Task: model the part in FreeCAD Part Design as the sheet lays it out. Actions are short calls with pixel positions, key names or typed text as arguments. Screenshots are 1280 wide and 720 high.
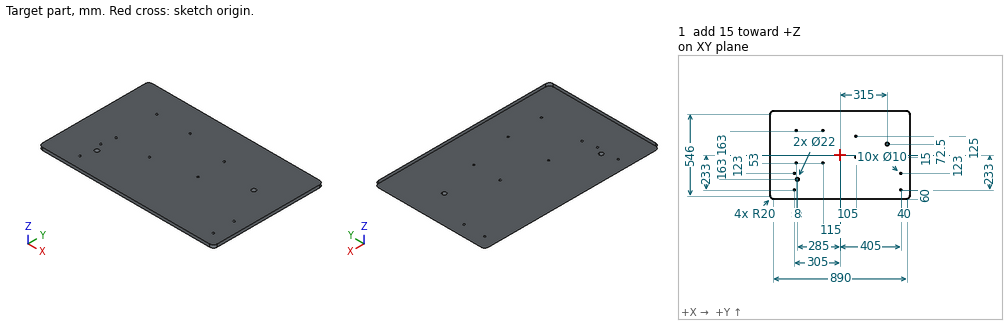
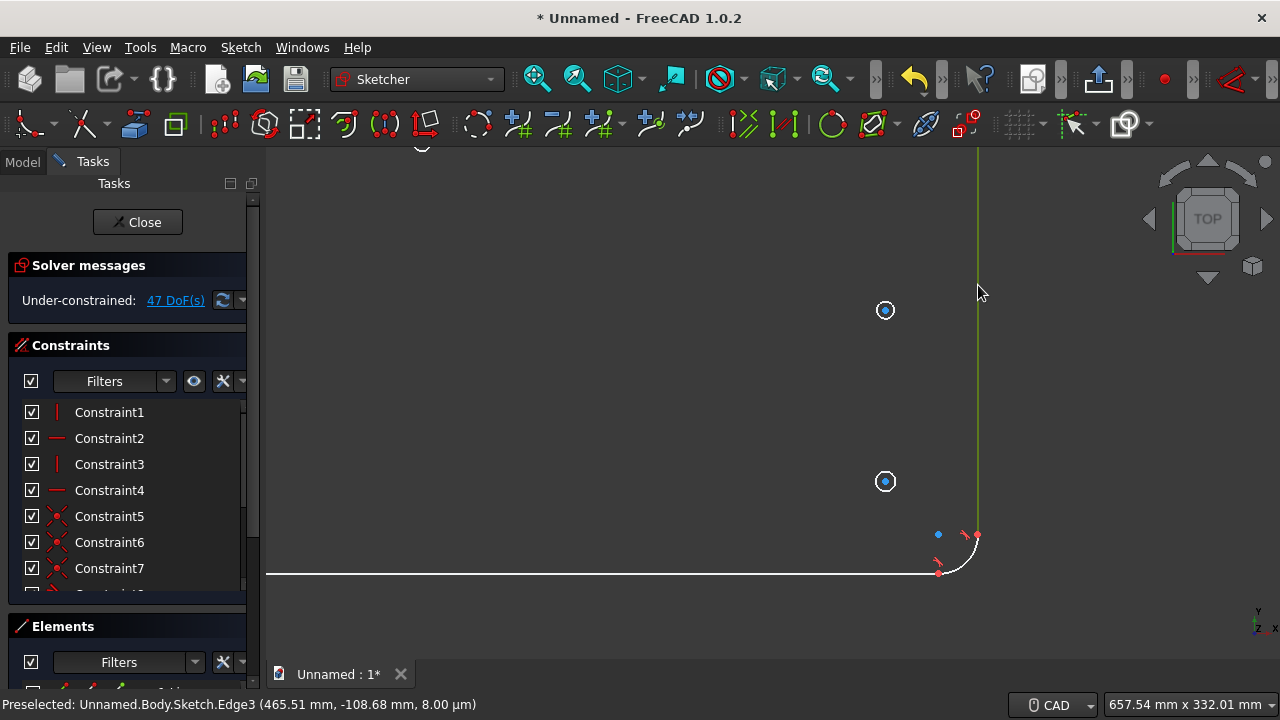
scroll(963, 569, down, 5)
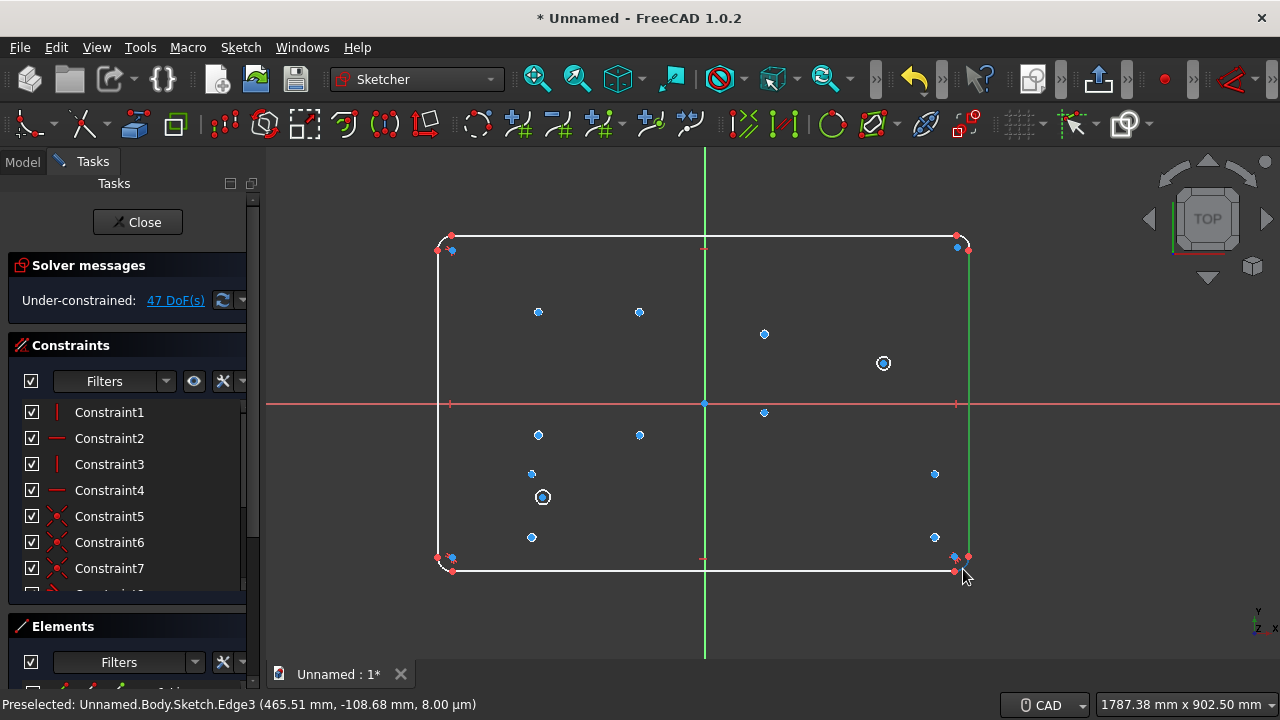
scroll(969, 244, up, 4)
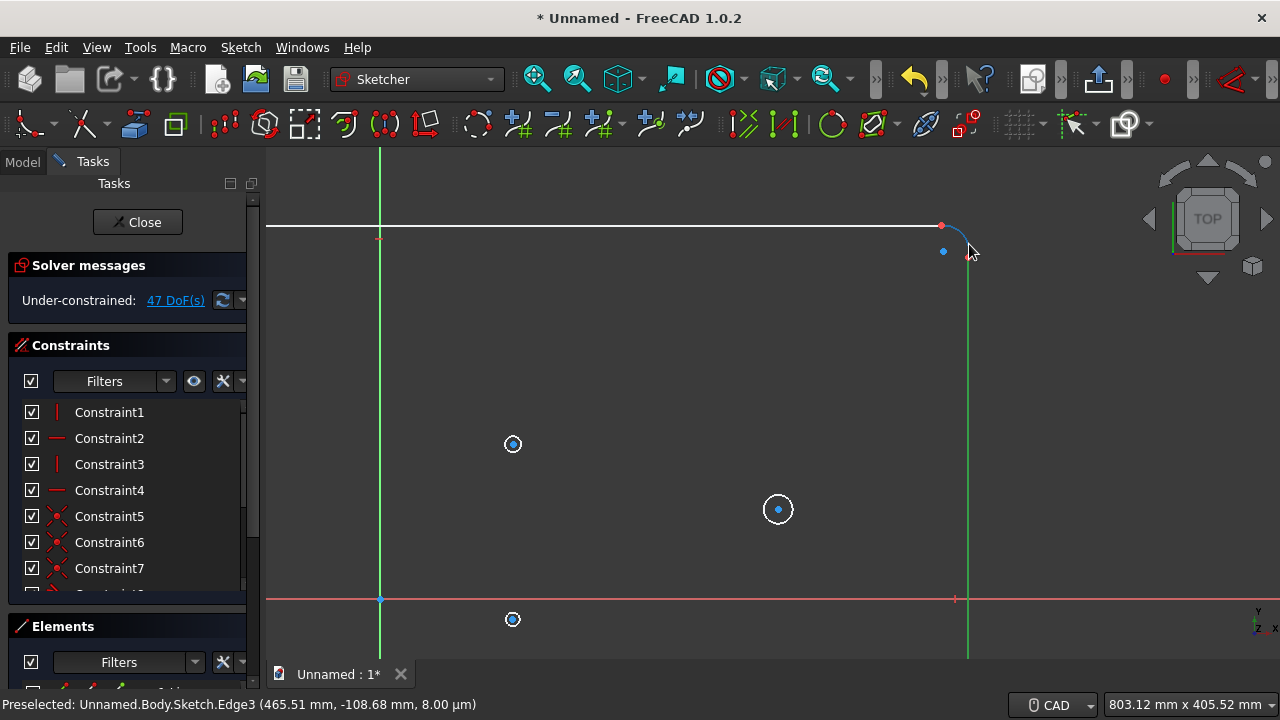
click(968, 243)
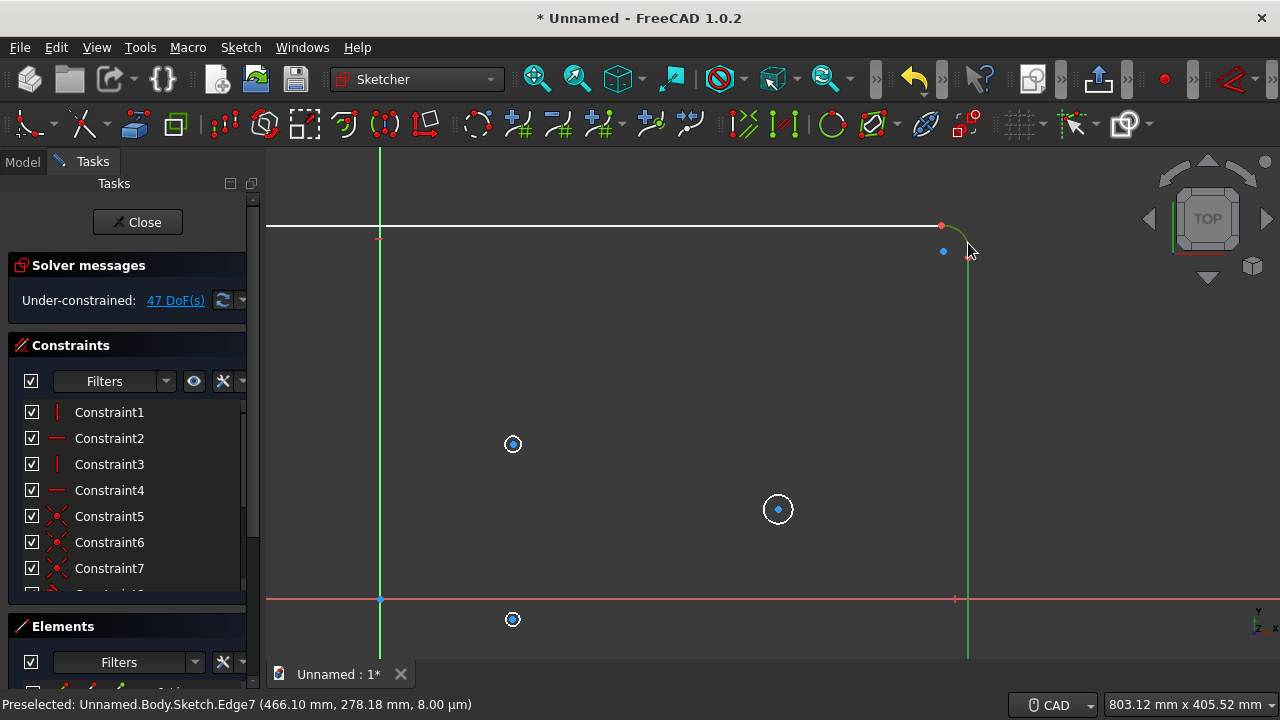
key(t)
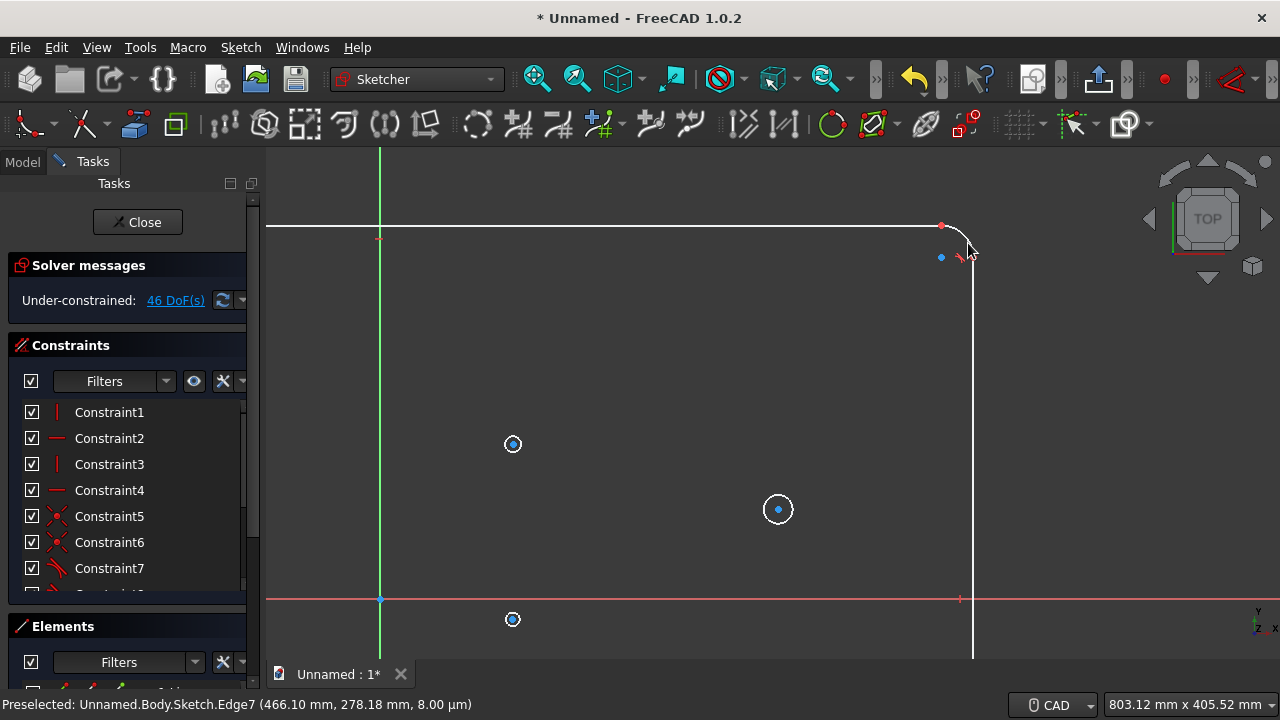
click(604, 226)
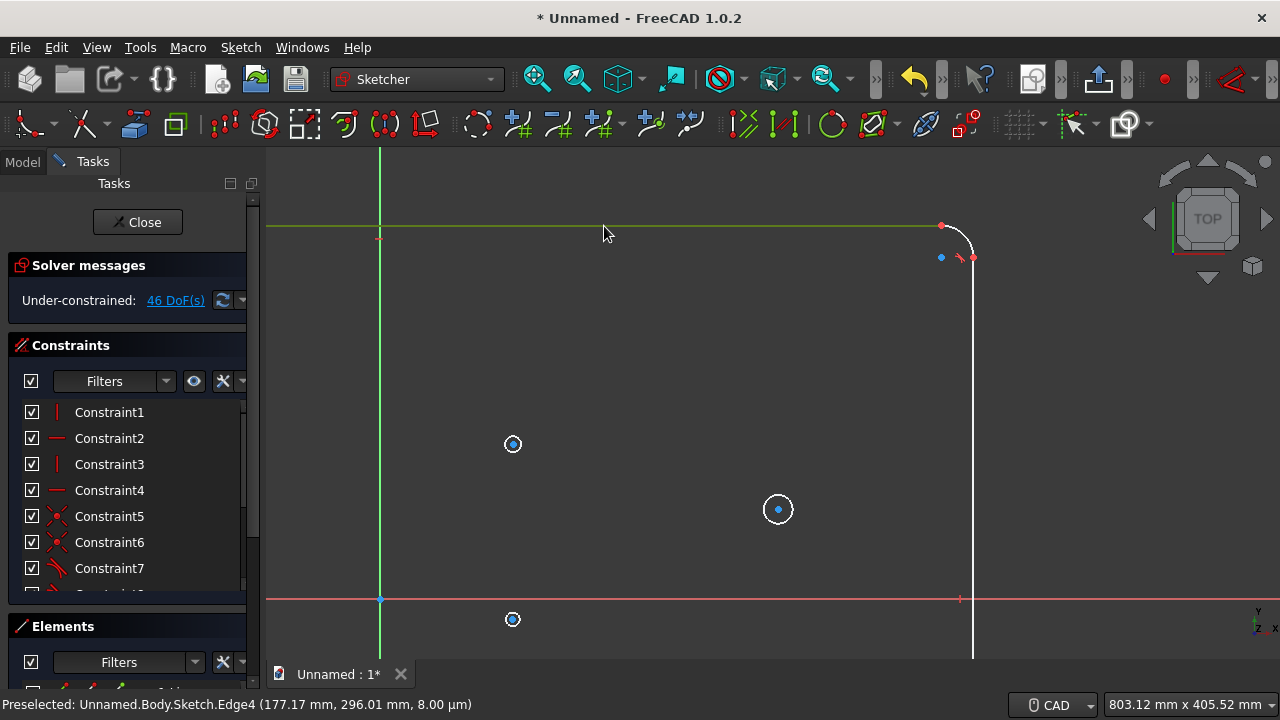
click(970, 243)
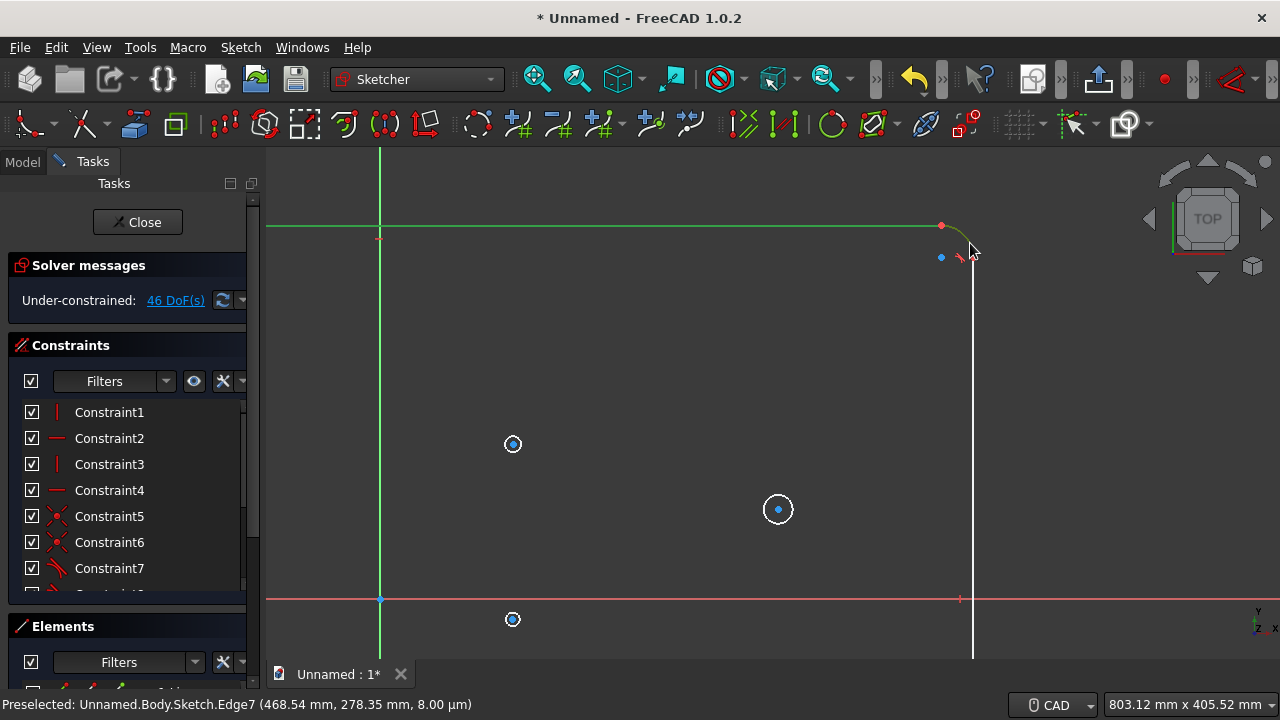
key(t)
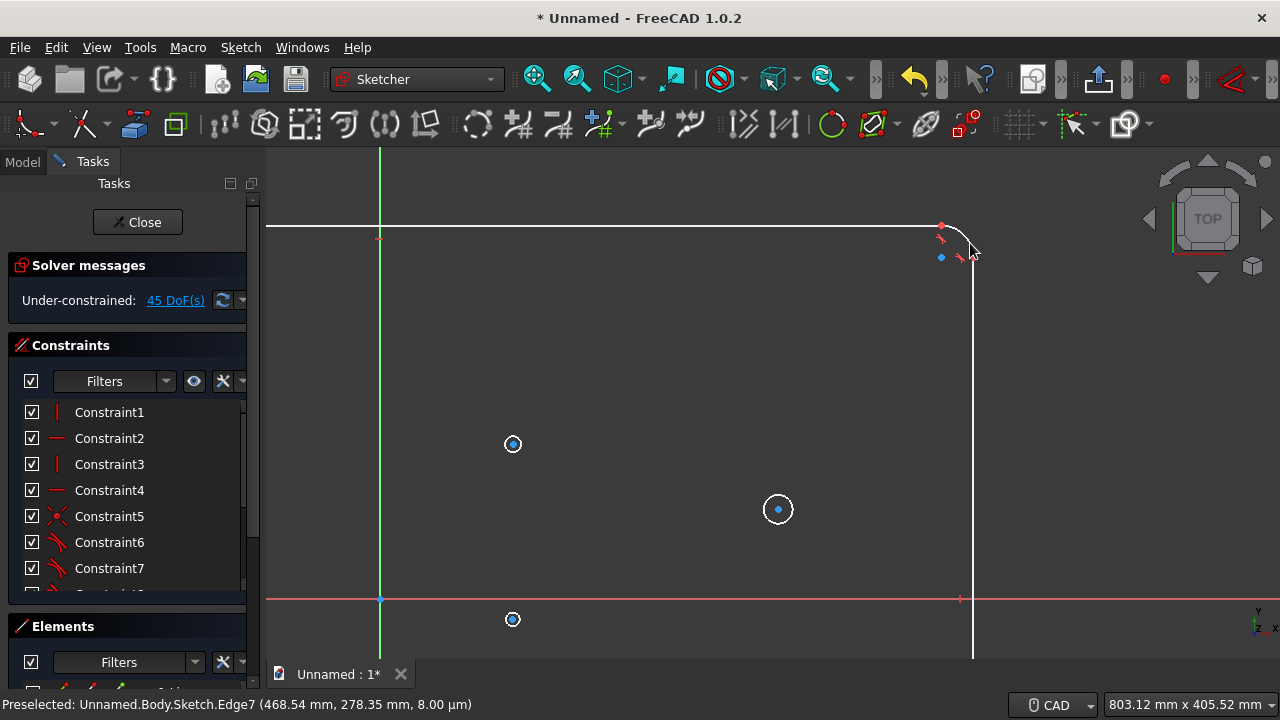
click(604, 226)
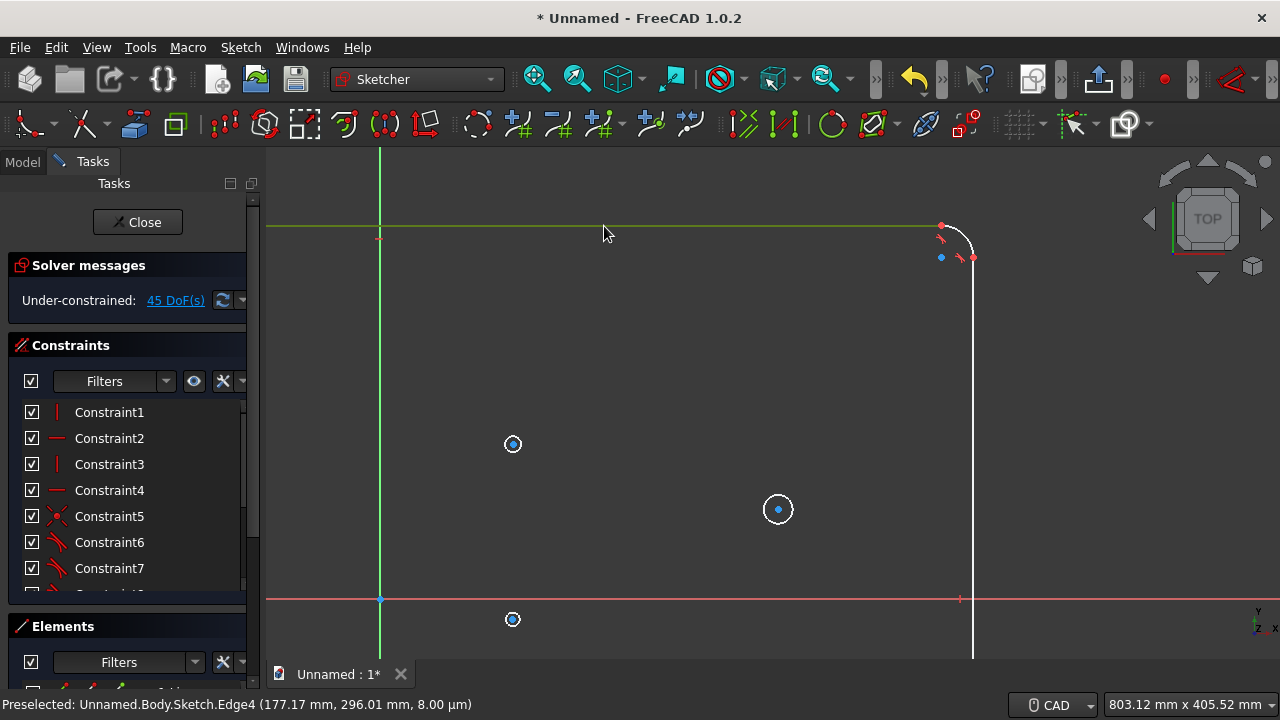
scroll(969, 243, down, 4)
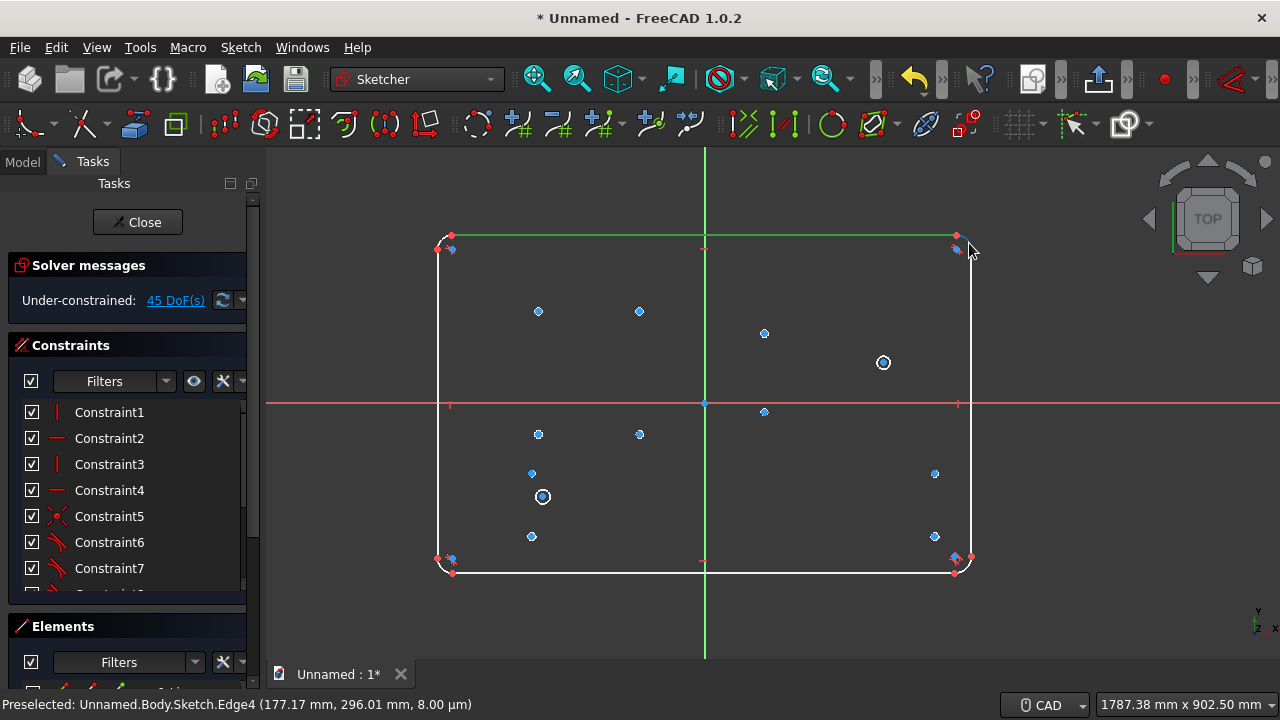
scroll(446, 237, up, 4)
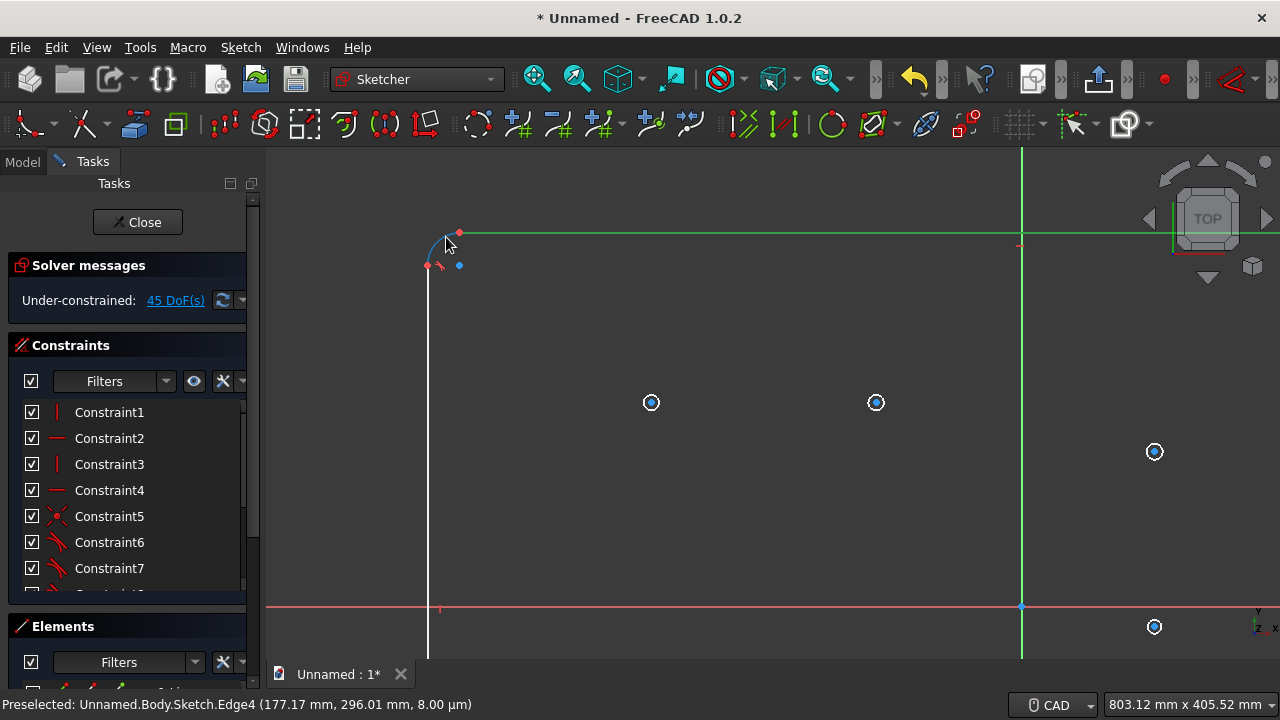
click(445, 237)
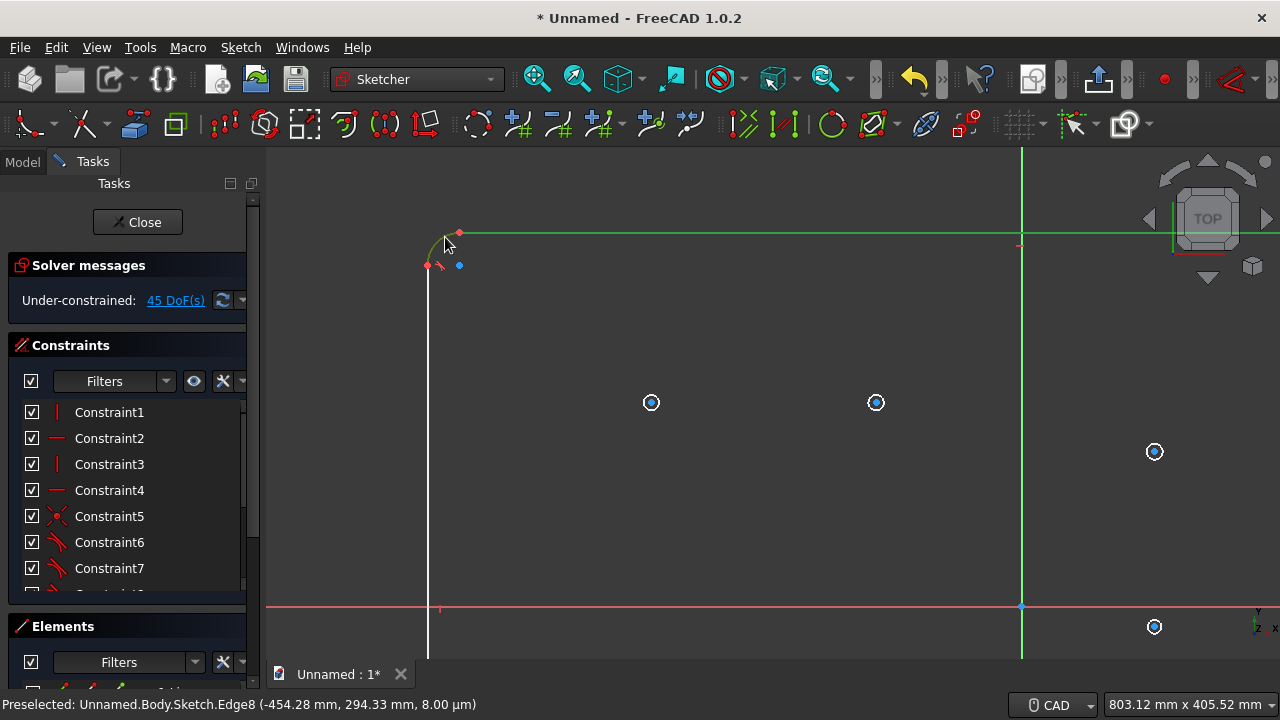
key(t)